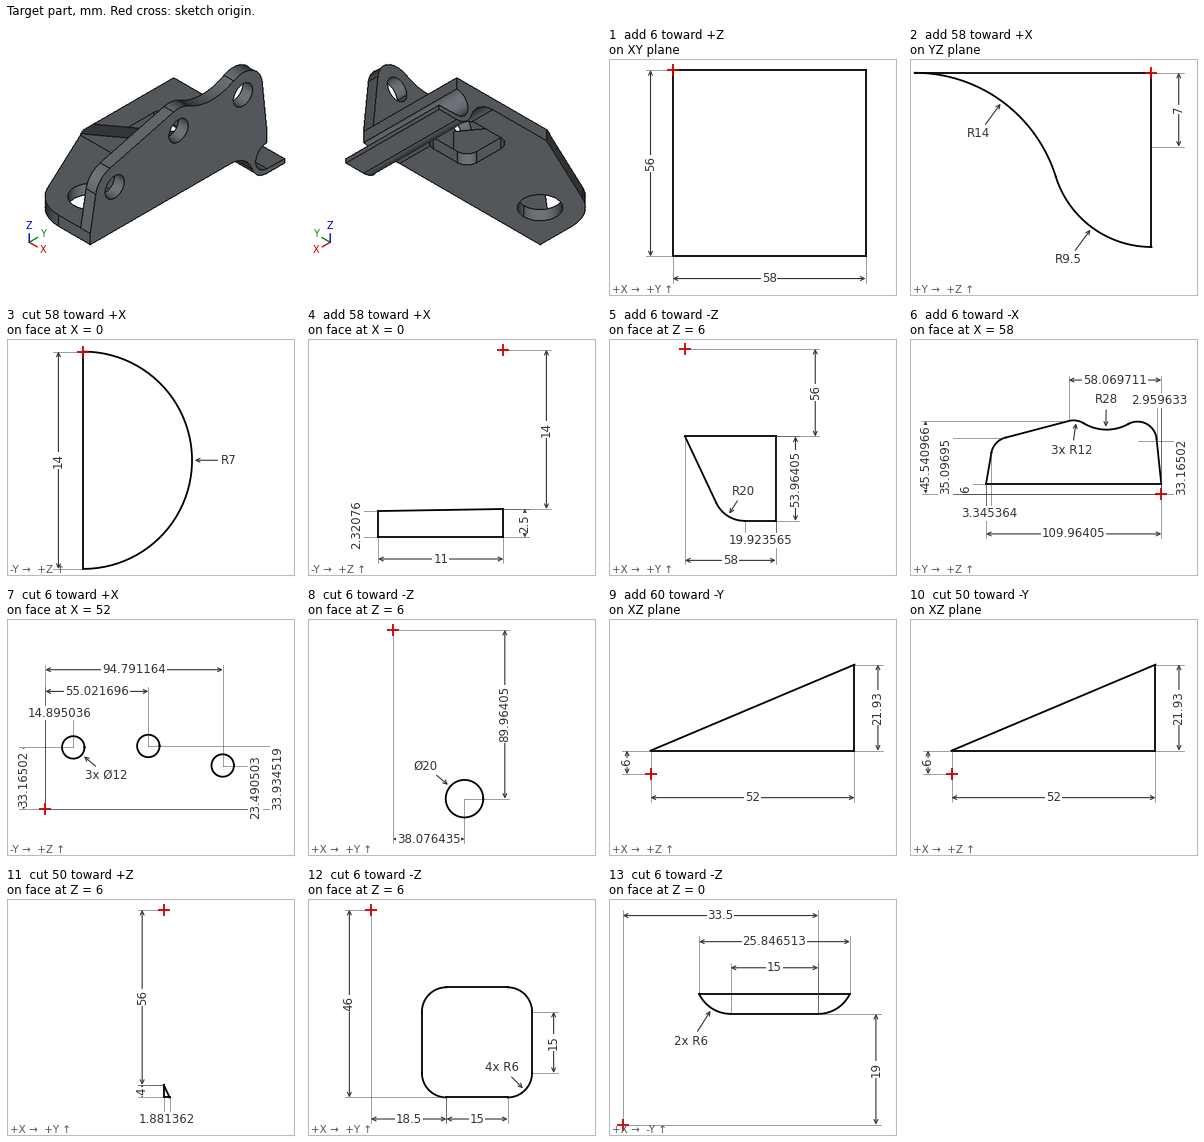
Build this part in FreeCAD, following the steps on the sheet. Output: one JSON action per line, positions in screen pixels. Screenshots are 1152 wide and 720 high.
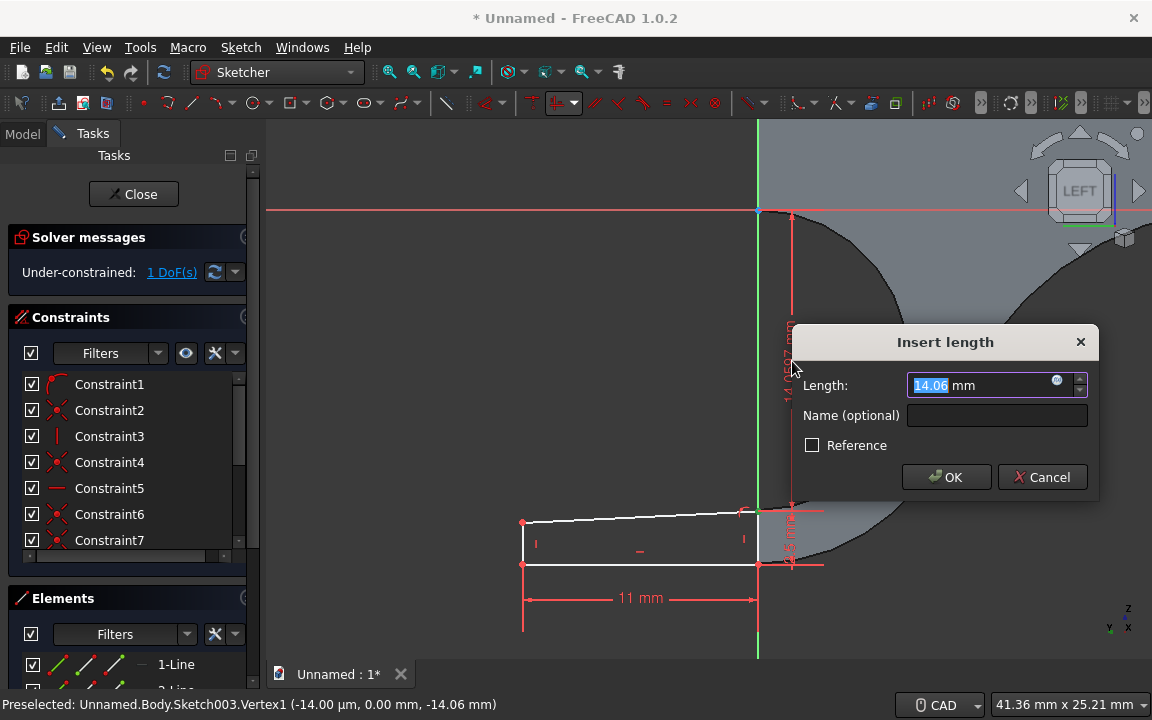
{"action": "type", "text": "14"}
{"action": "key", "text": "Return"}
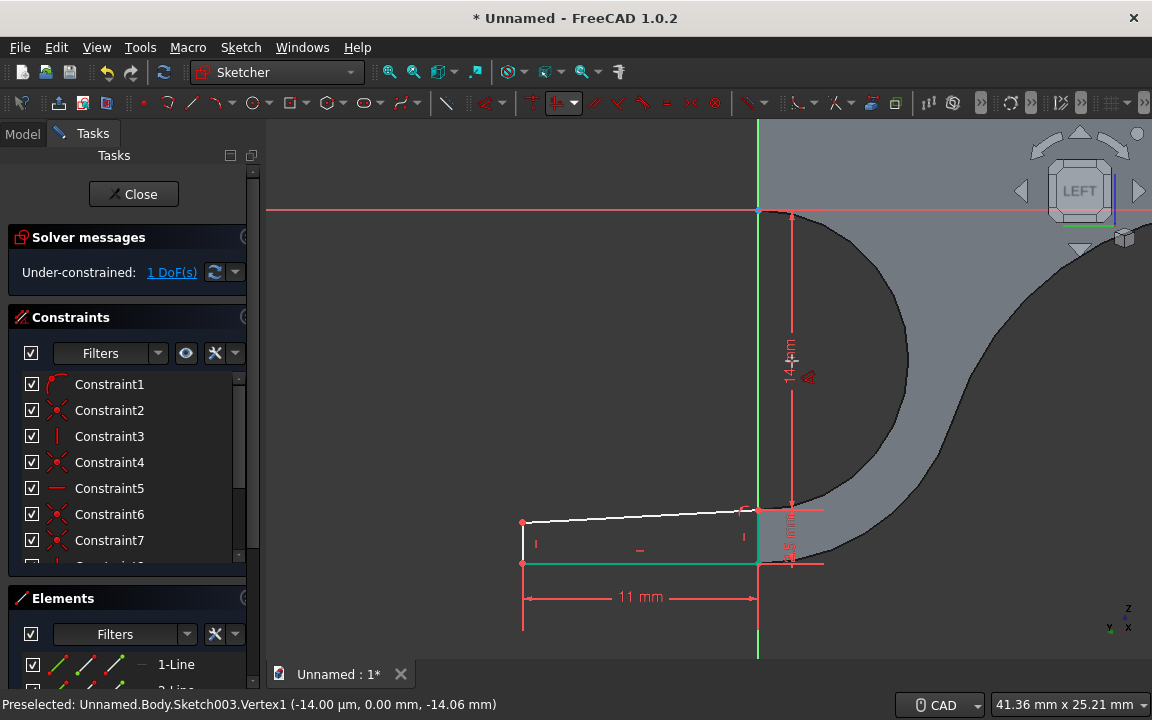
{"action": "left_click", "coordinate": [523, 535]}
{"action": "left_click", "coordinate": [489, 543]}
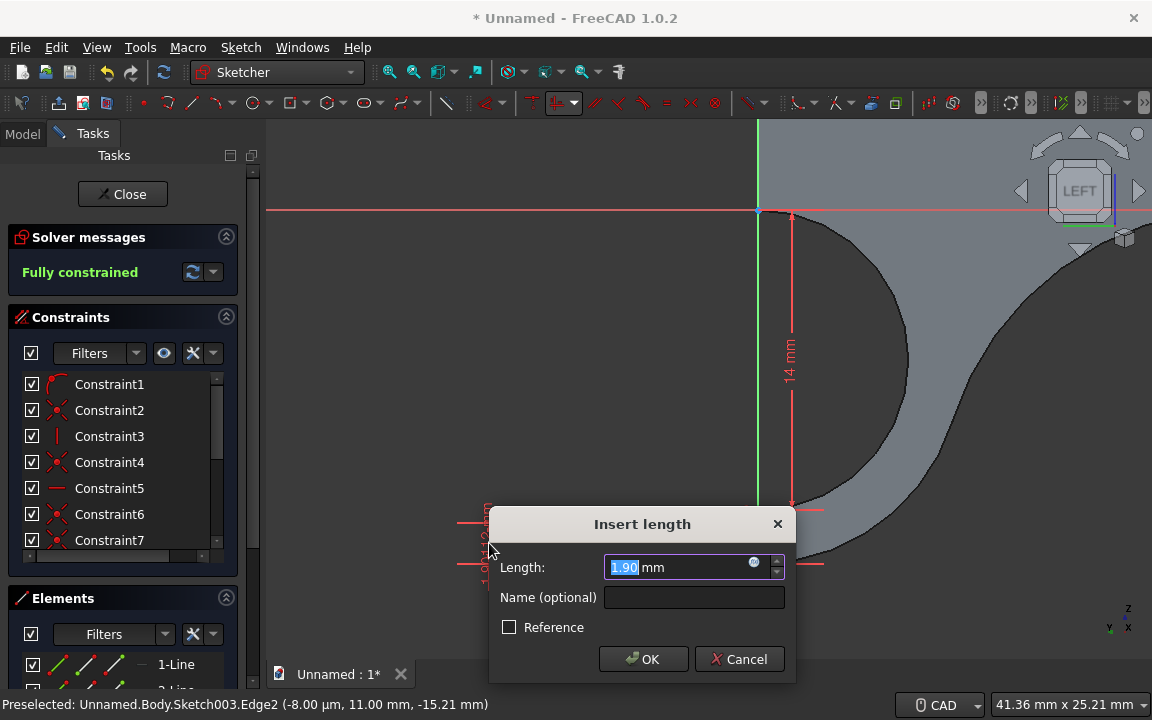
{"action": "type", "text": "2.32076"}
{"action": "key", "text": "Return"}
{"action": "key", "text": "Escape"}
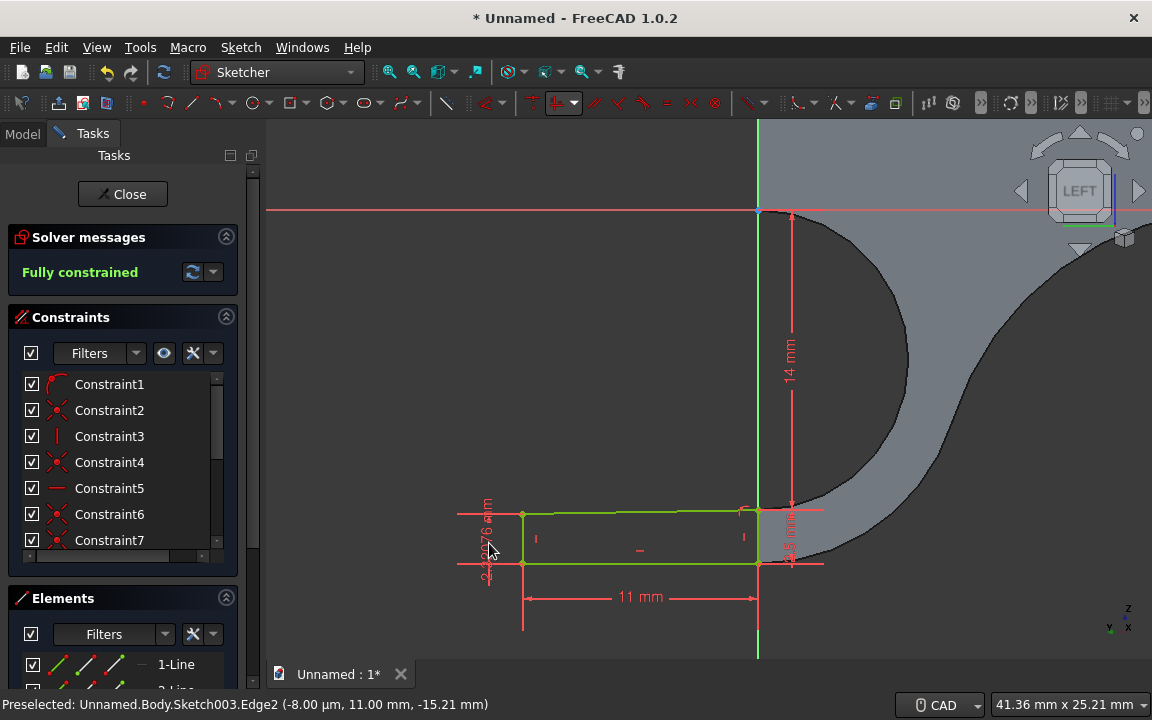
{"action": "left_click", "coordinate": [123, 194]}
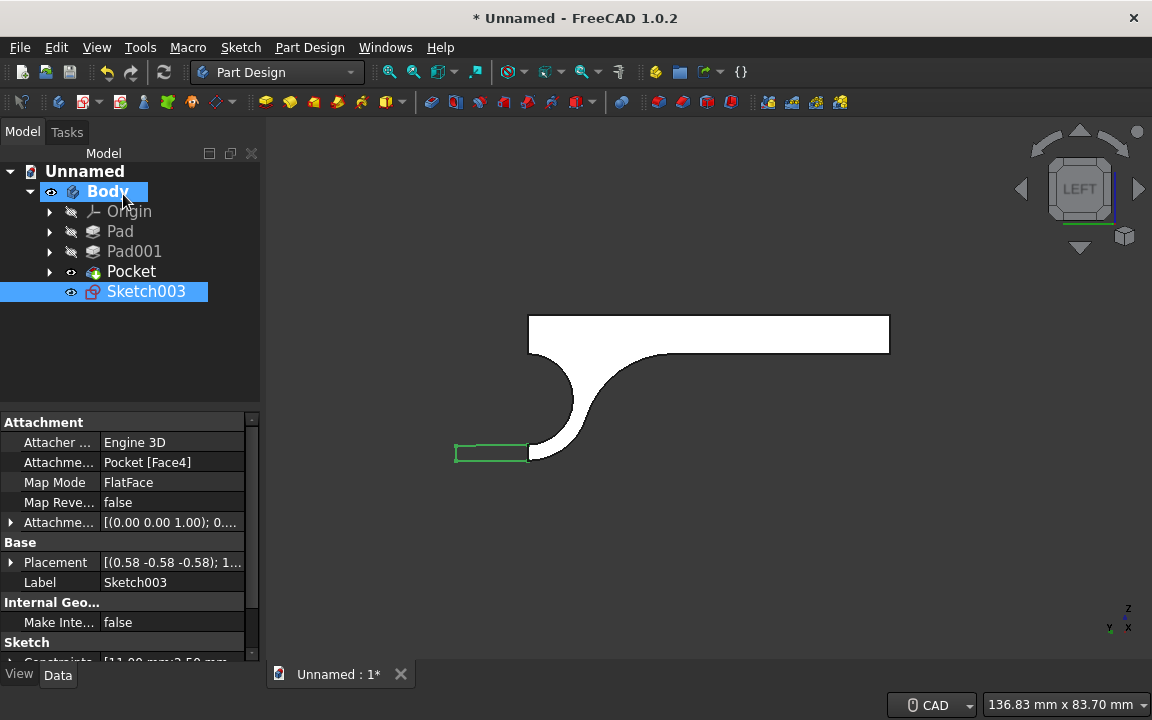
{"action": "left_click", "coordinate": [266, 102]}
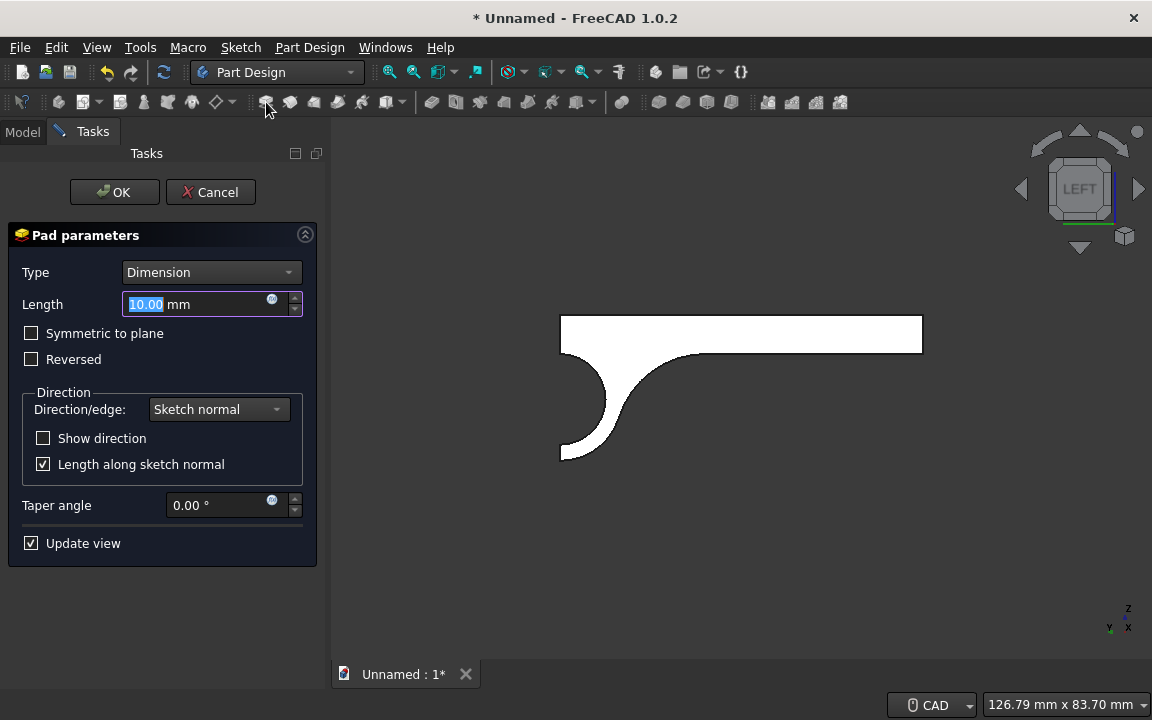
{"action": "type", "text": "58"}
{"action": "key", "text": "Tab"}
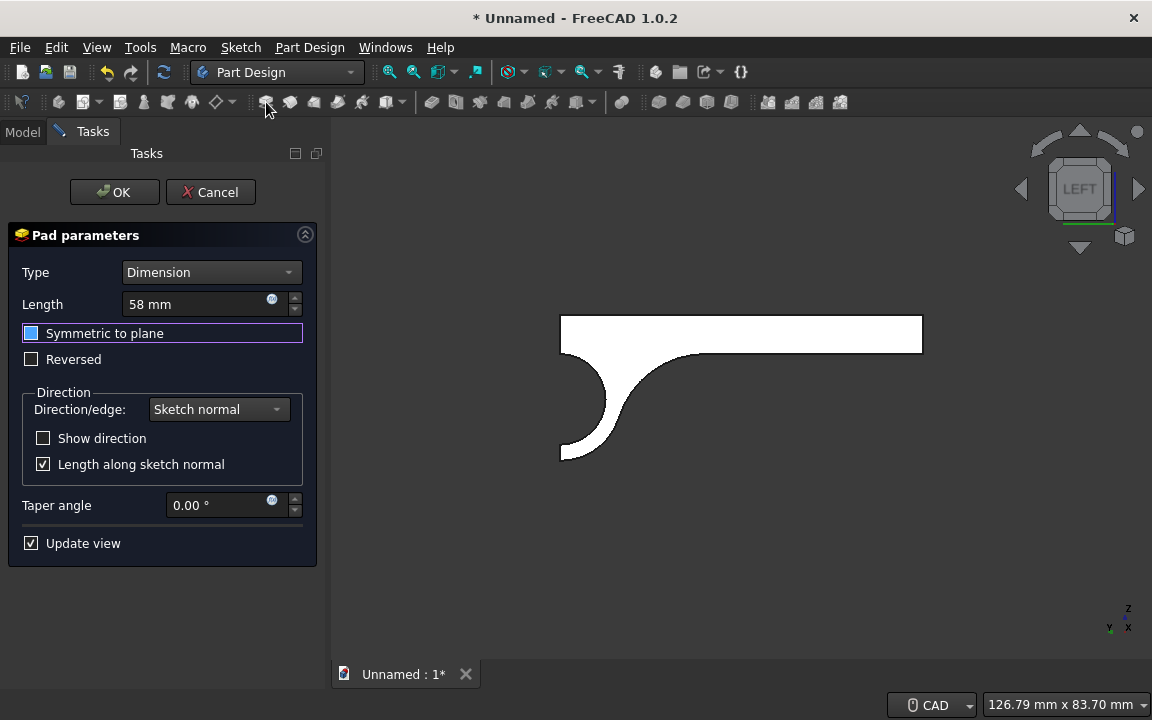
{"action": "left_click", "coordinate": [30, 359]}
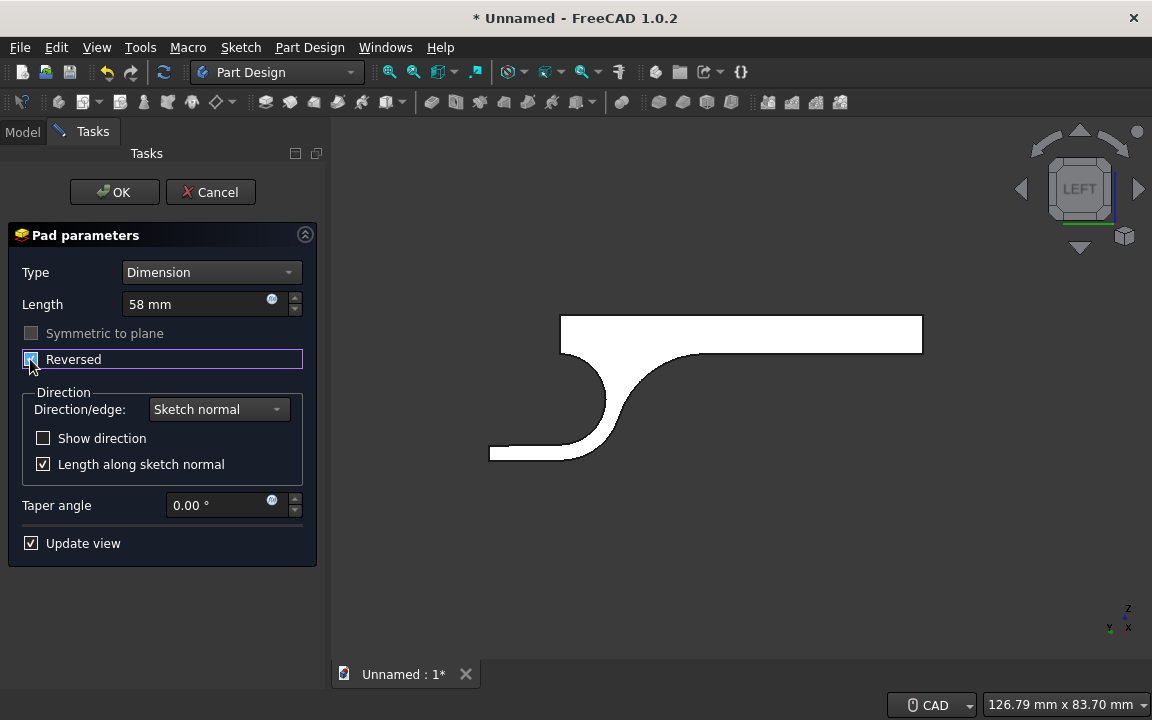
{"action": "left_click", "coordinate": [115, 192]}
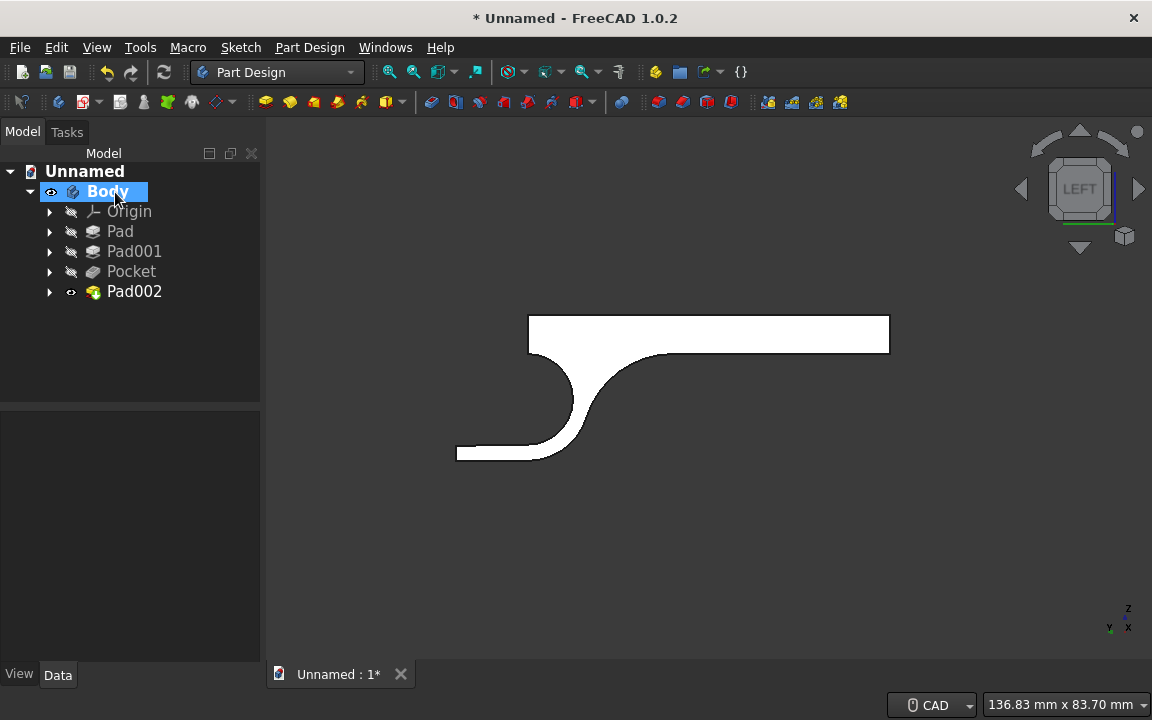
{"action": "key", "text": "0"}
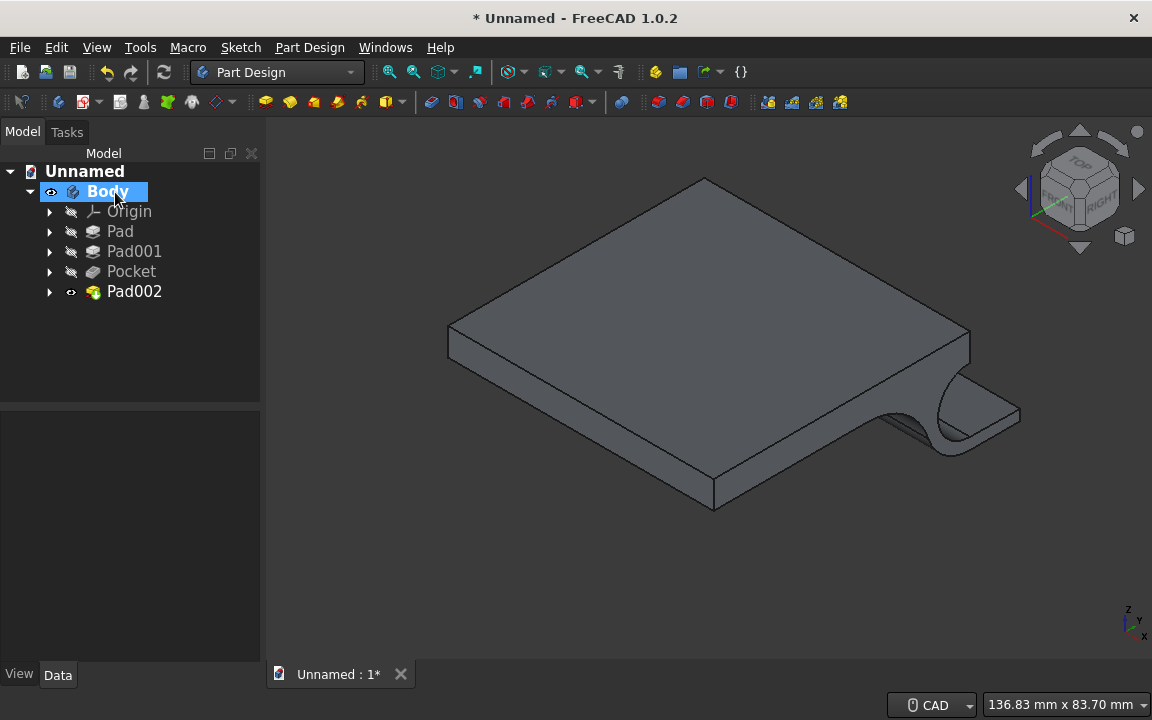
{"action": "left_click", "coordinate": [709, 328]}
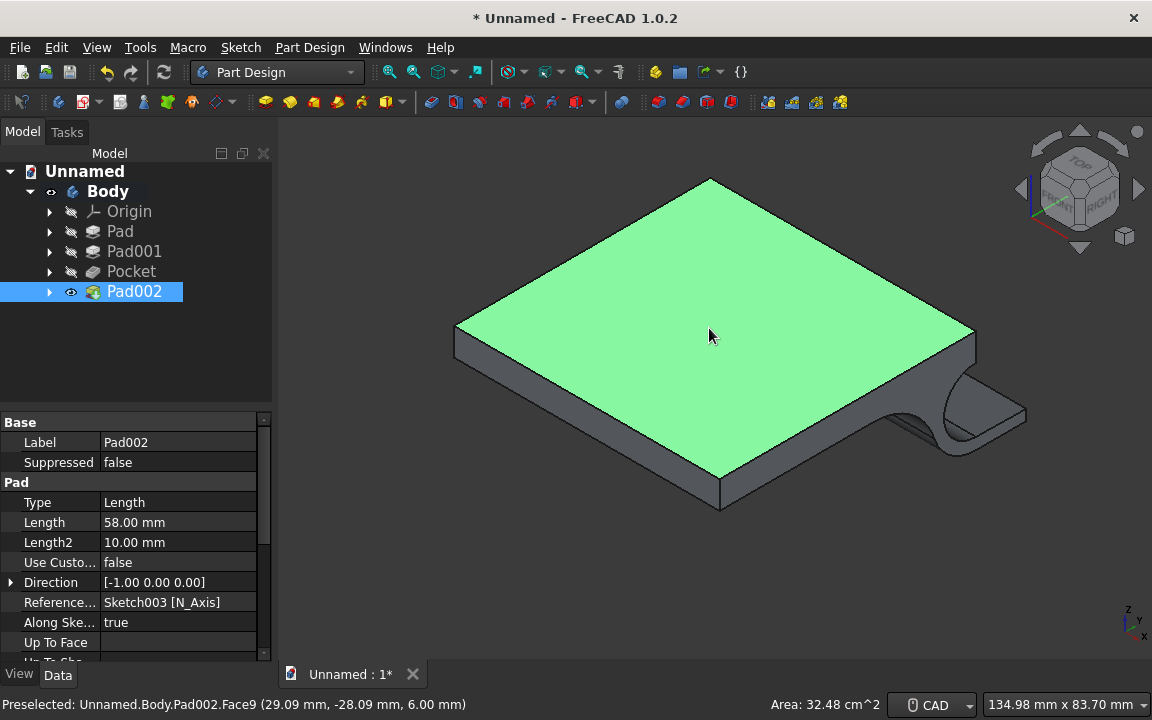
{"action": "left_click", "coordinate": [84, 102]}